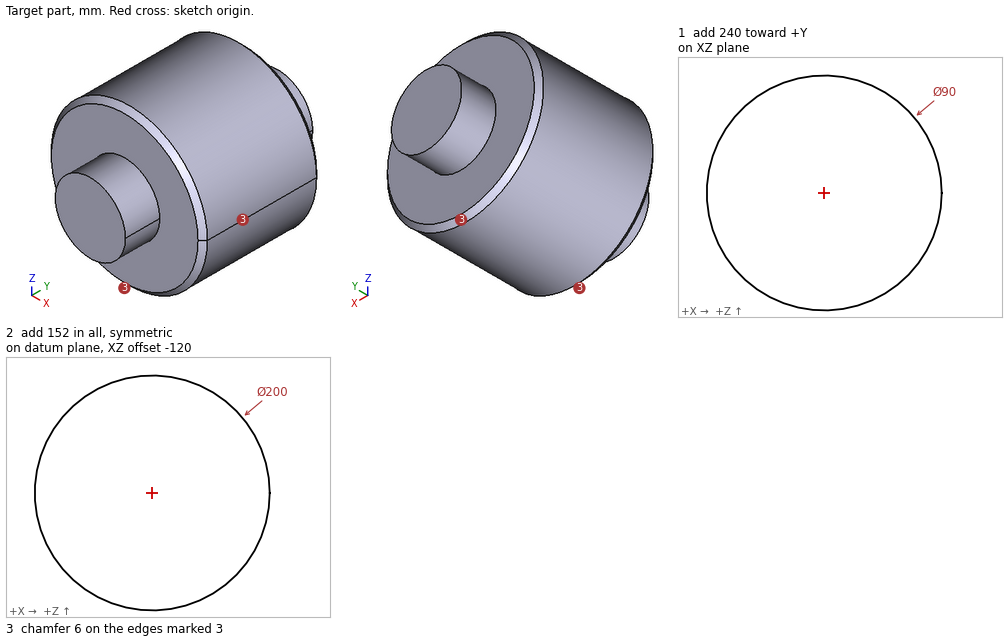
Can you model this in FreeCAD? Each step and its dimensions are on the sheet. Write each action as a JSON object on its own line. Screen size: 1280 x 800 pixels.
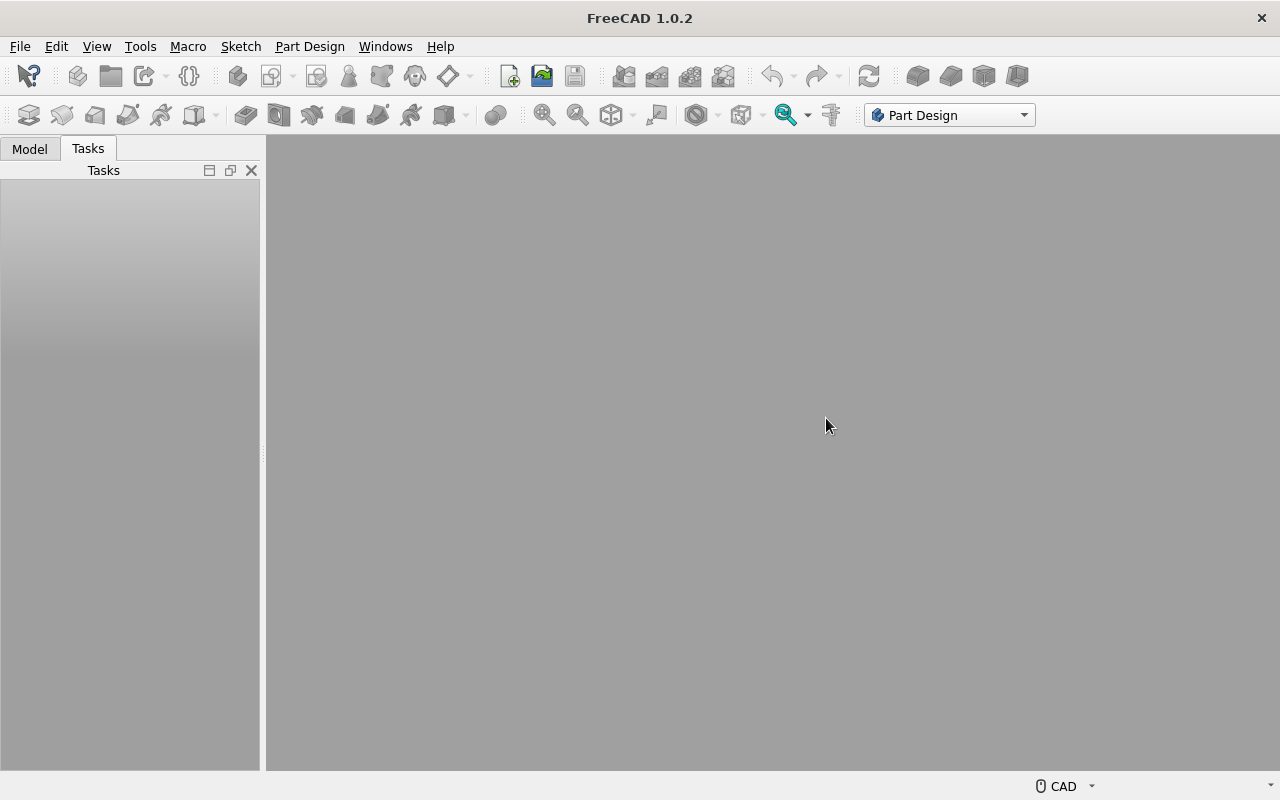
{"action": "key", "text": "ctrl+n"}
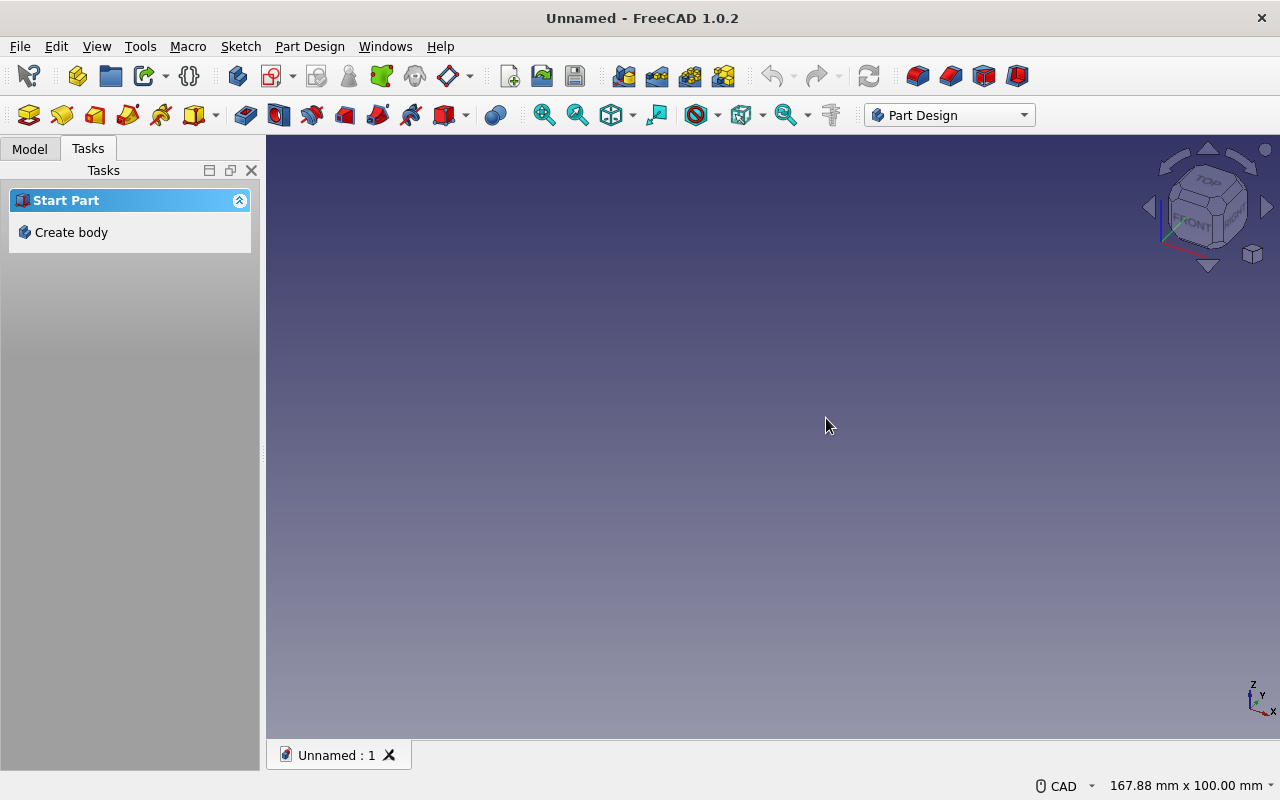
{"action": "left_click", "coordinate": [270, 76]}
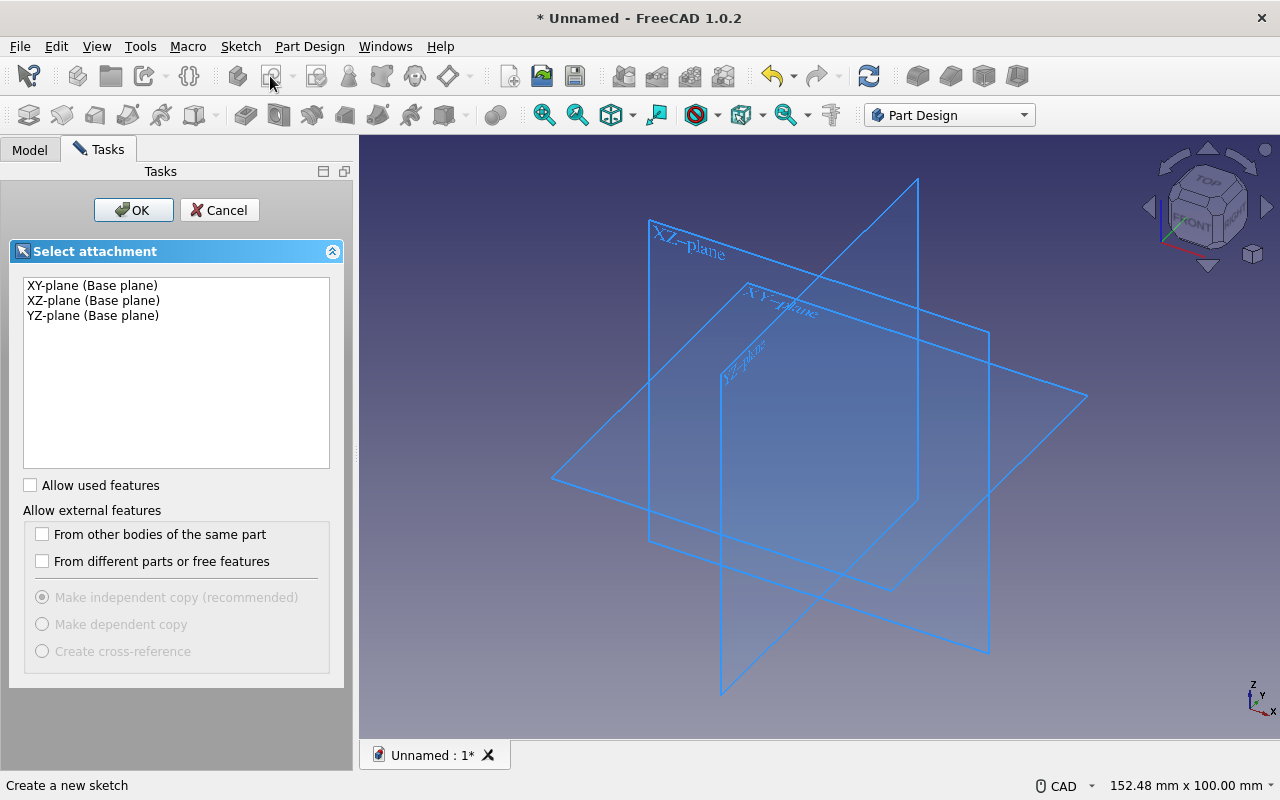
{"action": "left_click", "coordinate": [84, 300]}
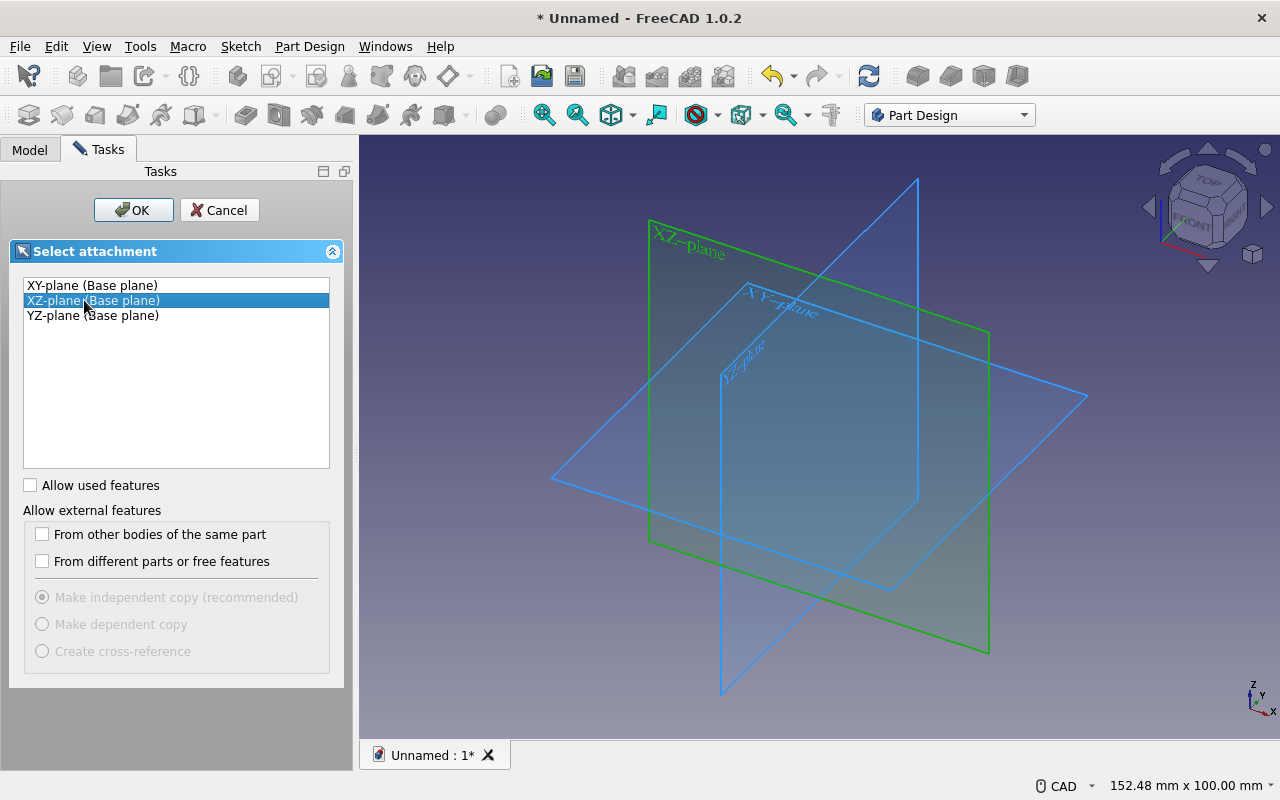
{"action": "left_click", "coordinate": [134, 210]}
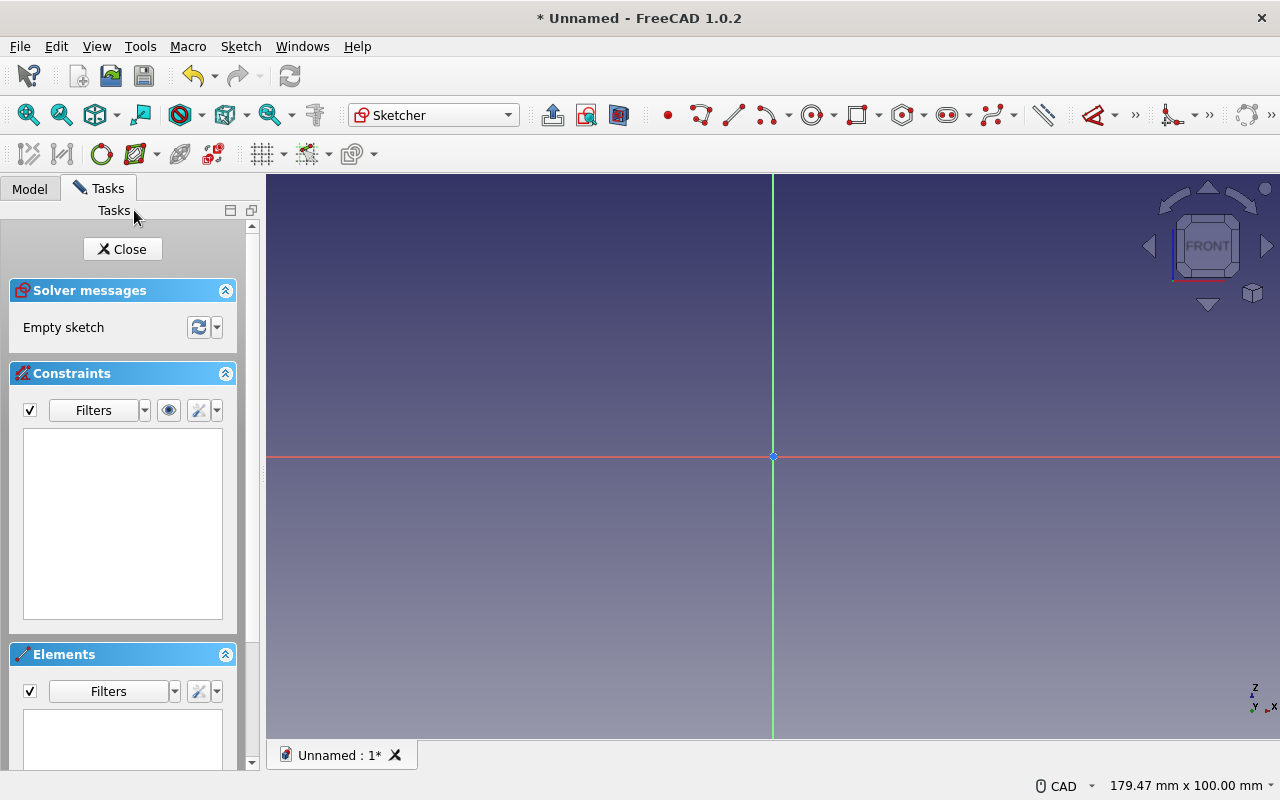
{"action": "scroll", "coordinate": [565, 457], "scroll_direction": "down", "scroll_amount": 2}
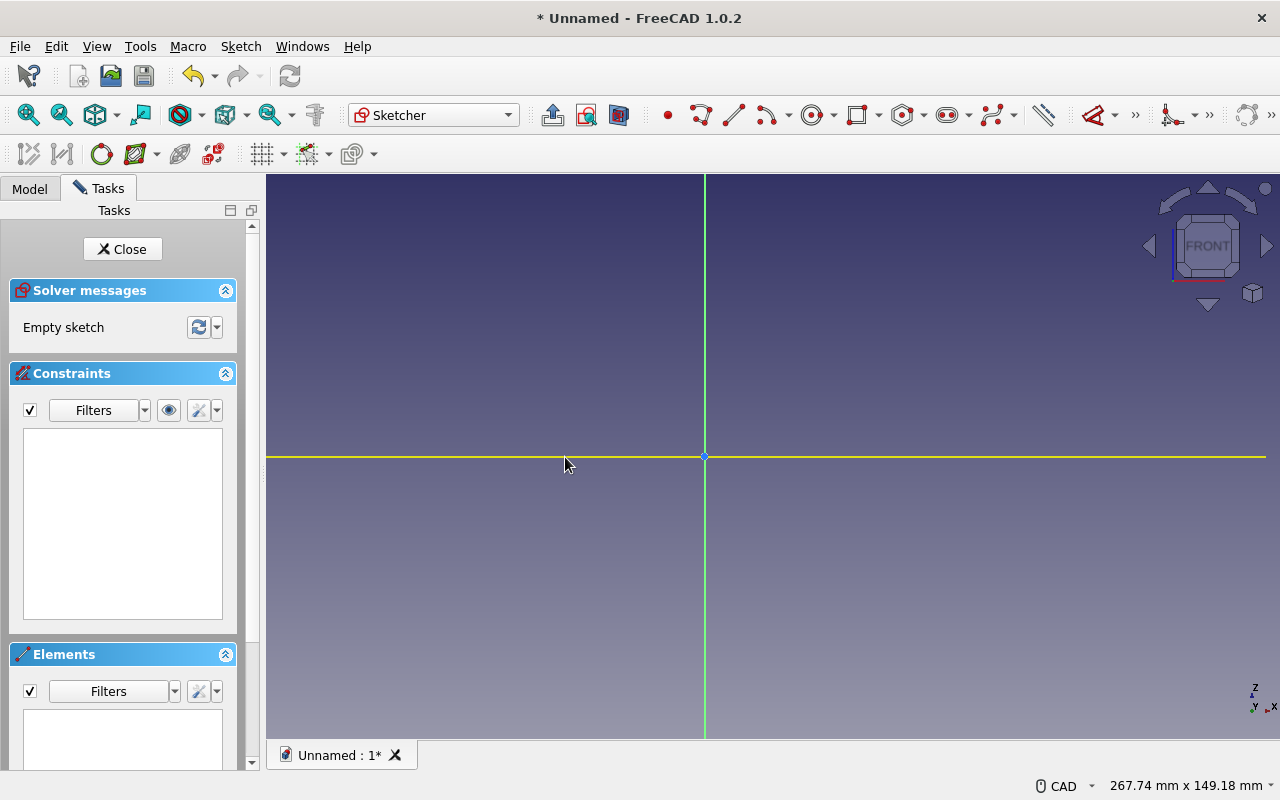
{"action": "key", "text": "g c"}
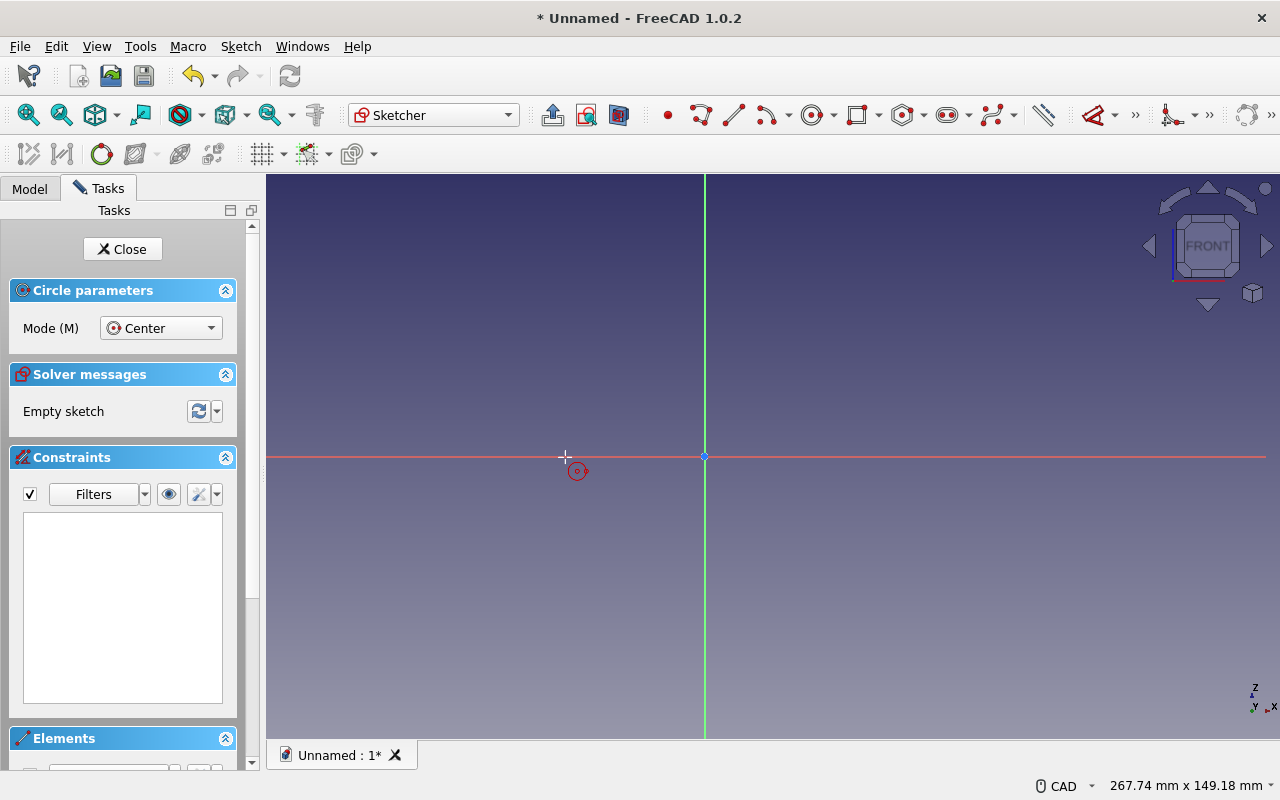
{"action": "left_click", "coordinate": [705, 457]}
{"action": "left_click", "coordinate": [825, 336]}
{"action": "key", "text": "Escape"}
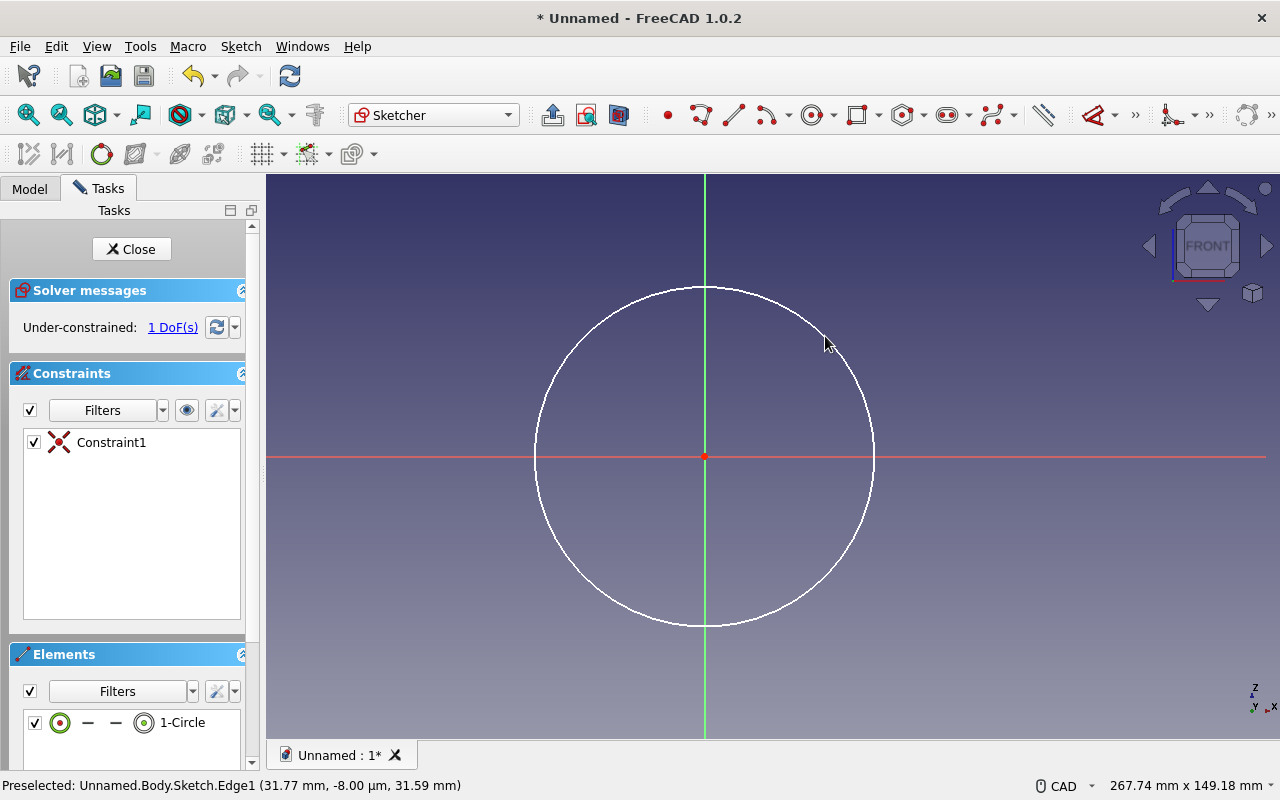
{"action": "left_click", "coordinate": [824, 336]}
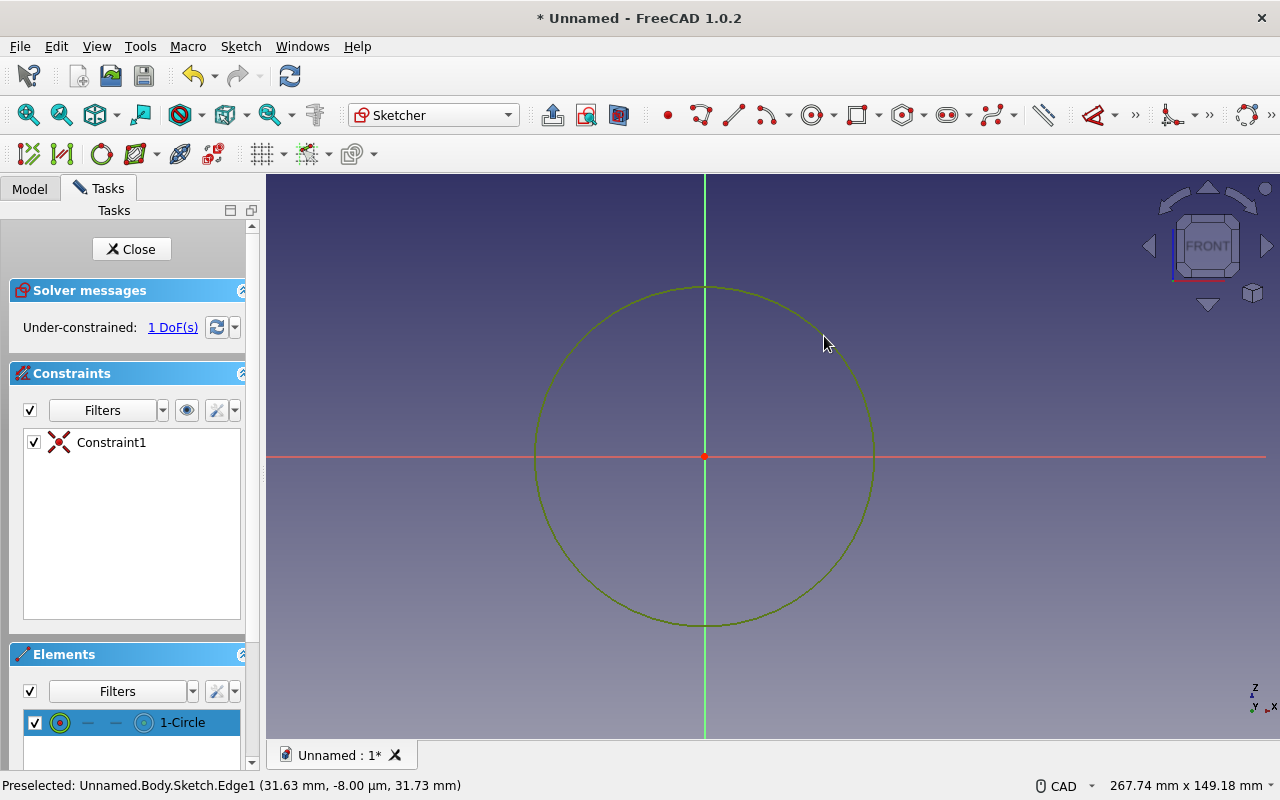
{"action": "left_click", "coordinate": [1114, 116]}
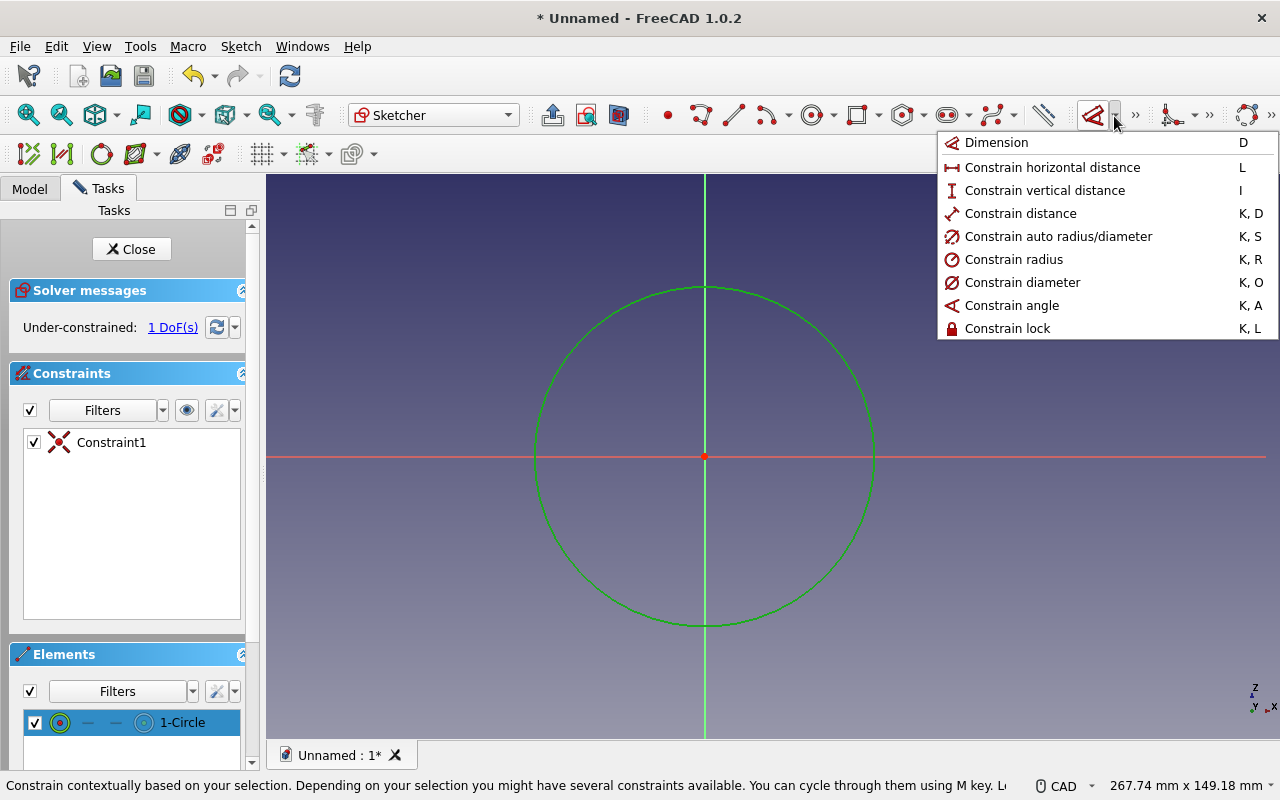
{"action": "left_click", "coordinate": [1108, 282]}